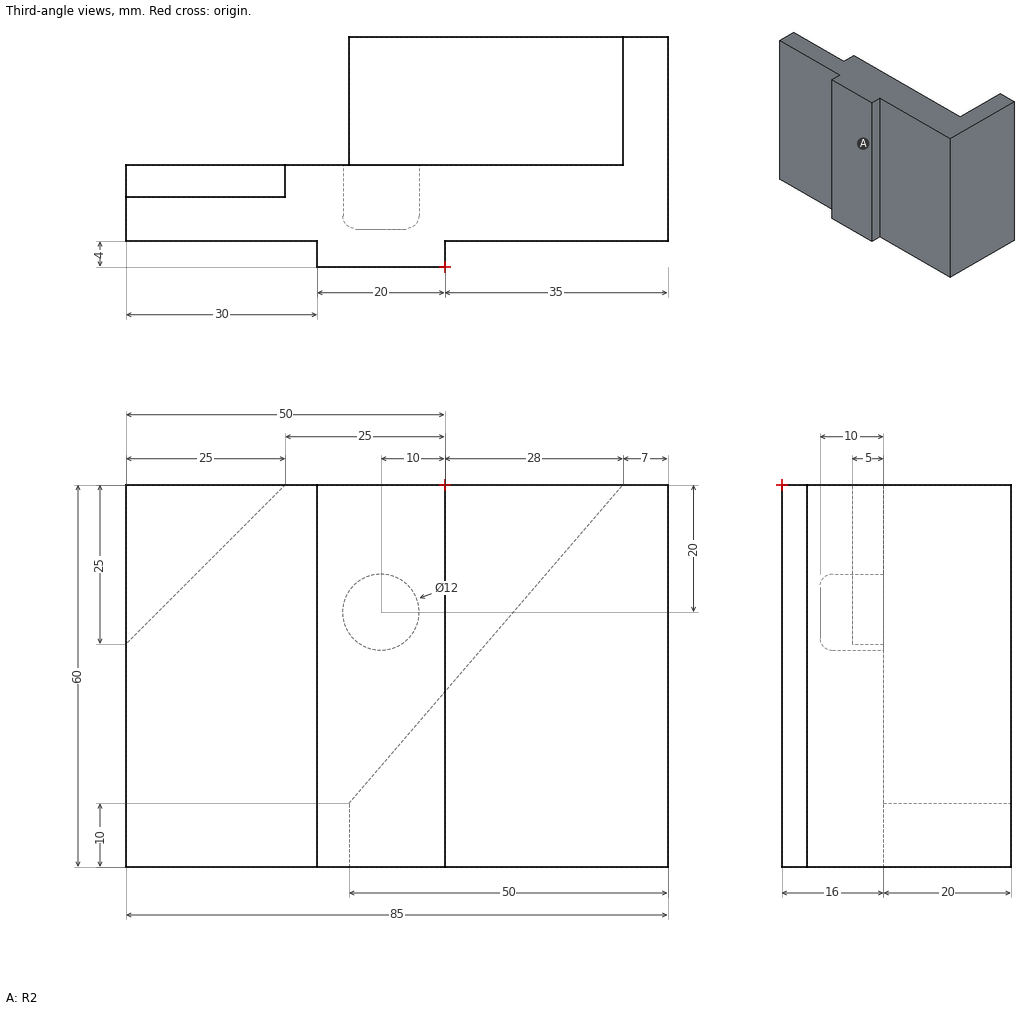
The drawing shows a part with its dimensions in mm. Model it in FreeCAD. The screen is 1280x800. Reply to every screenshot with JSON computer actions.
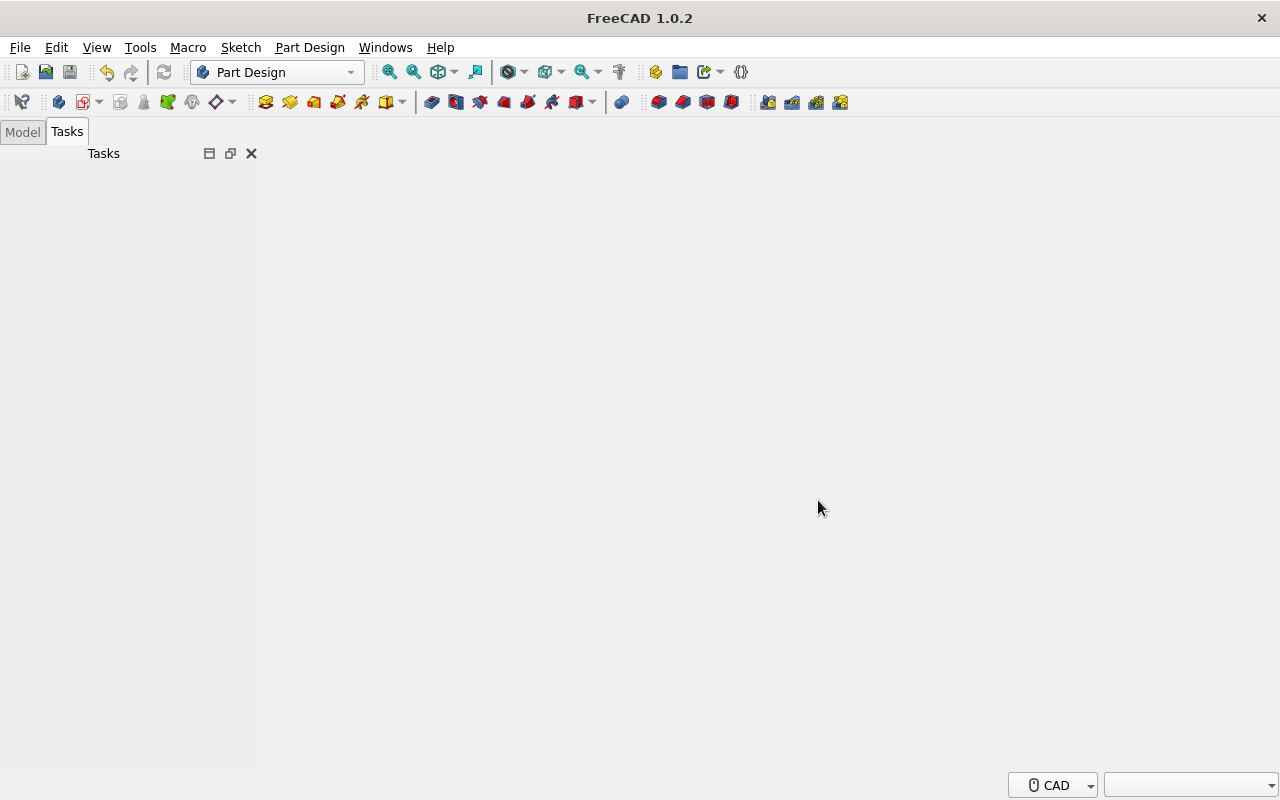
{"action": "left_click", "coordinate": [22, 72]}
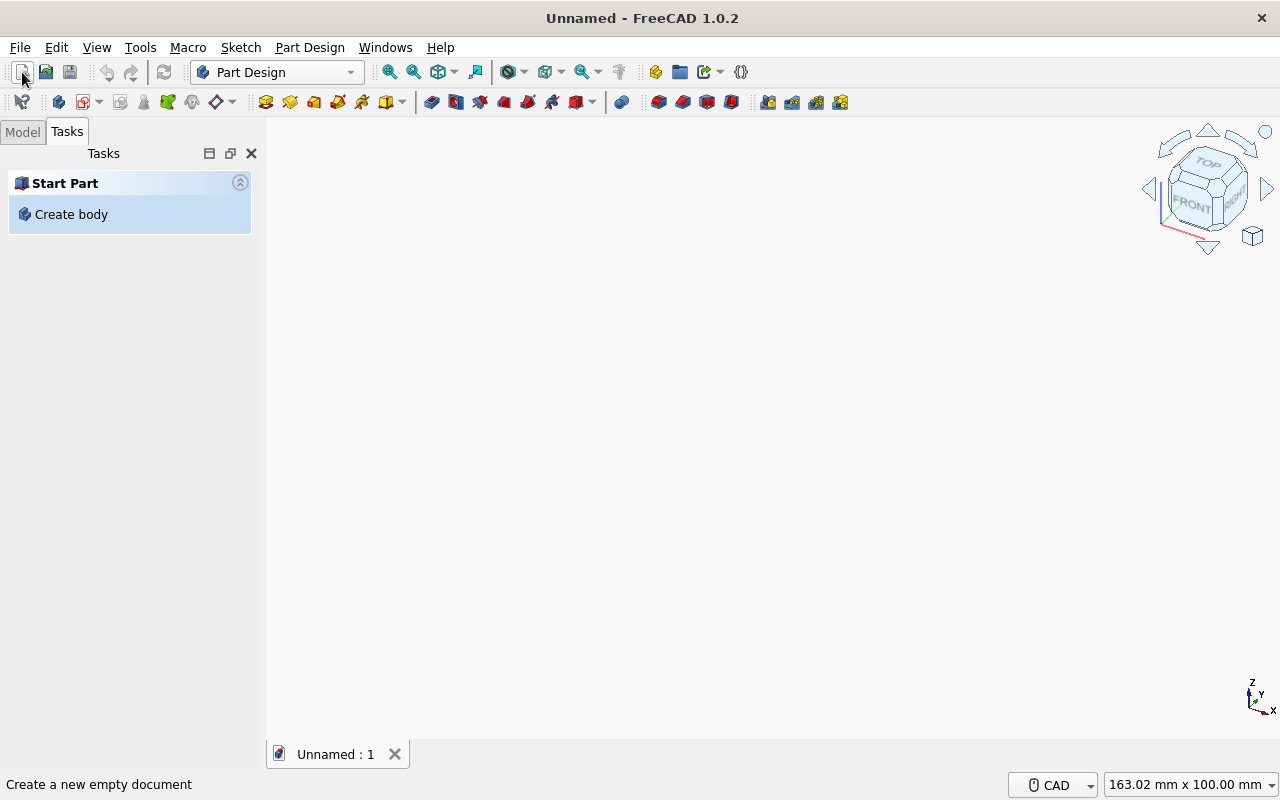
{"action": "left_click", "coordinate": [84, 102]}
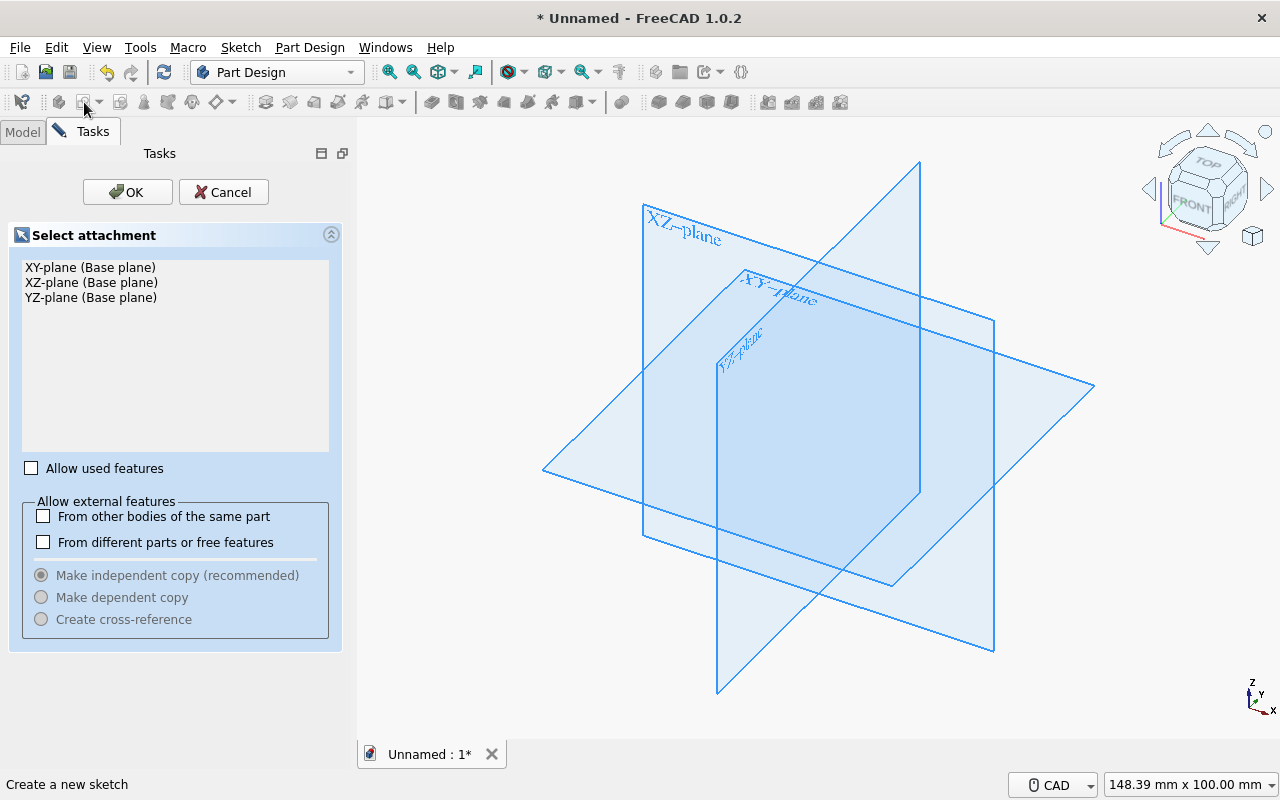
{"action": "left_click", "coordinate": [82, 282]}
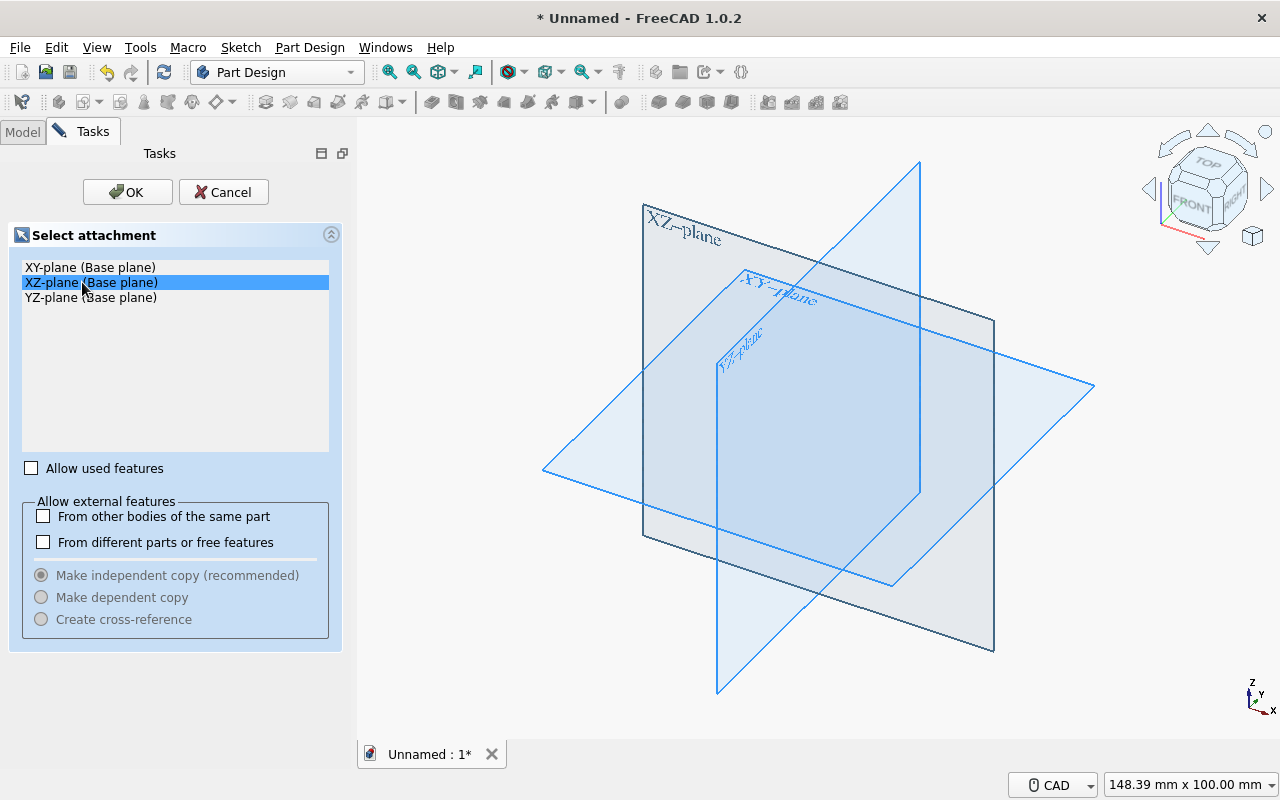
{"action": "left_click", "coordinate": [128, 192]}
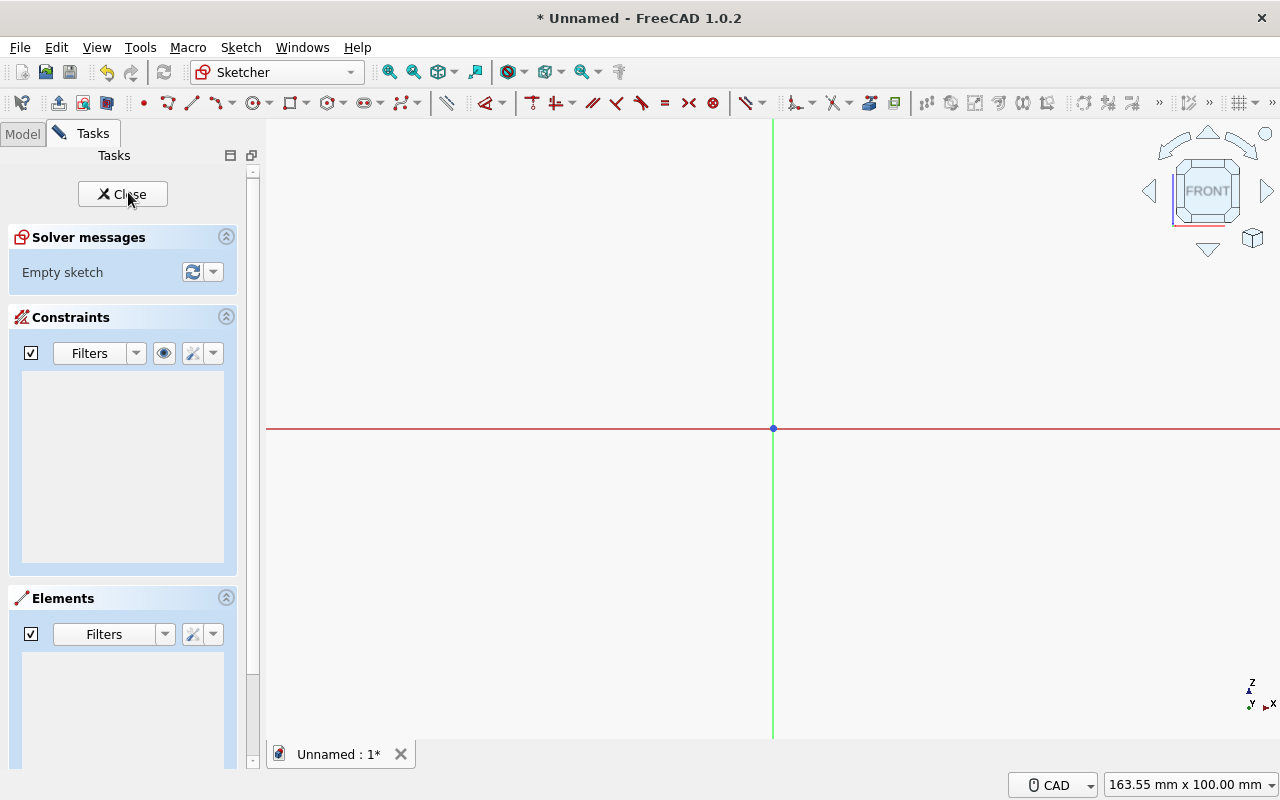
{"action": "scroll", "coordinate": [605, 147], "scroll_direction": "down", "scroll_amount": 1}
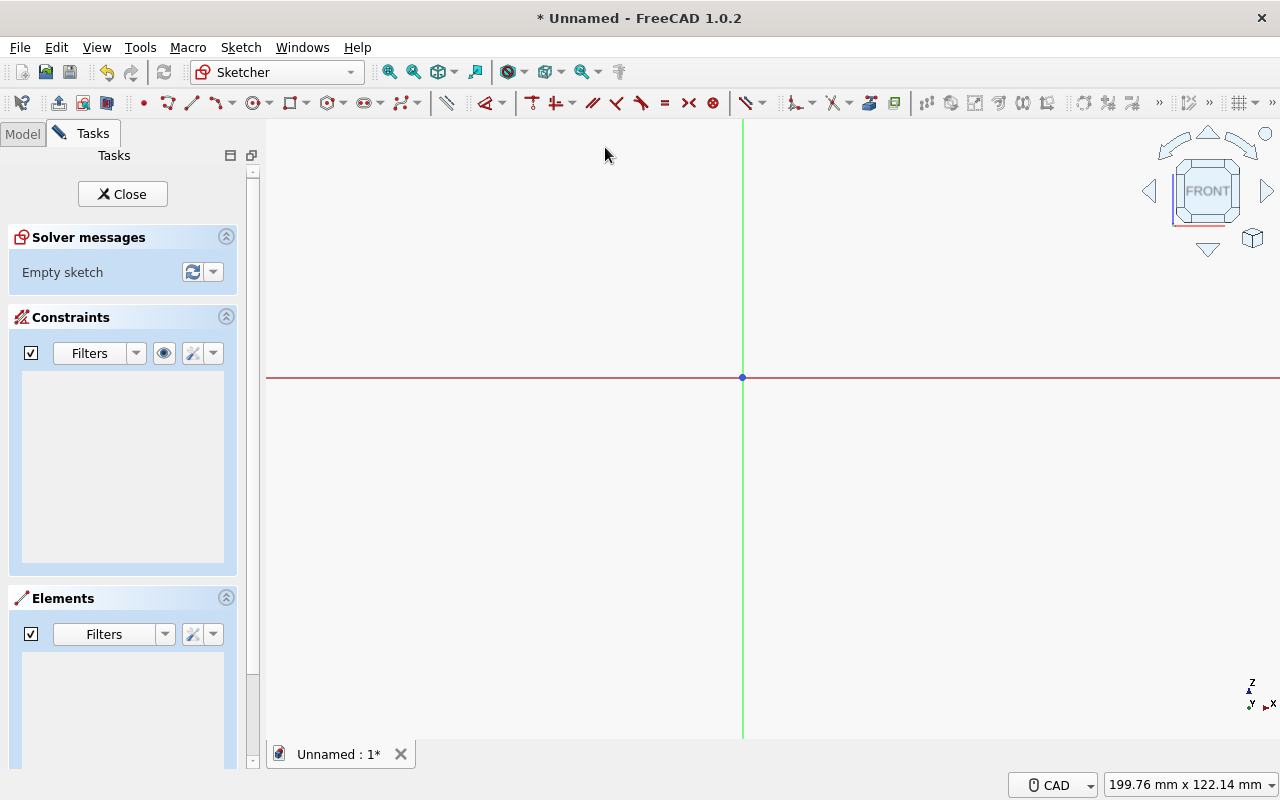
{"action": "left_click", "coordinate": [290, 104]}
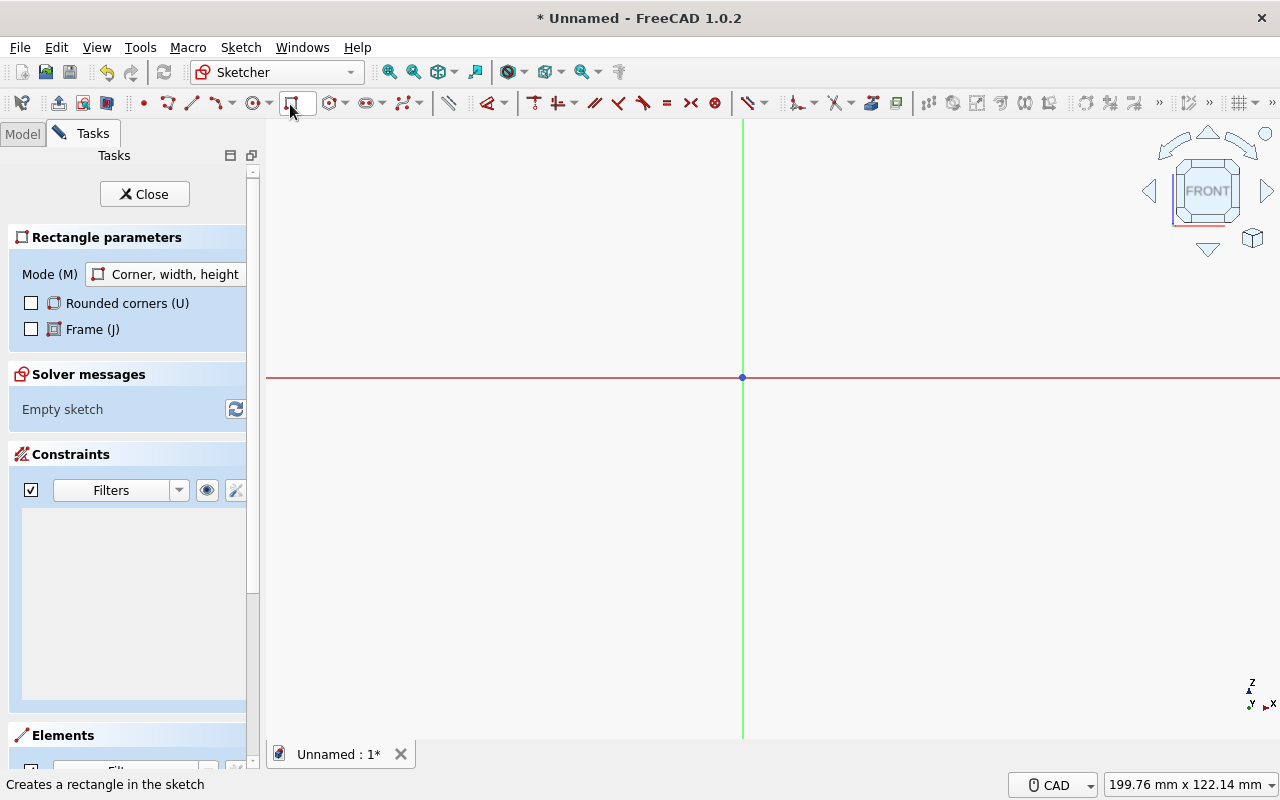
{"action": "left_click", "coordinate": [489, 378]}
{"action": "left_click", "coordinate": [920, 682]}
{"action": "key", "text": "Escape"}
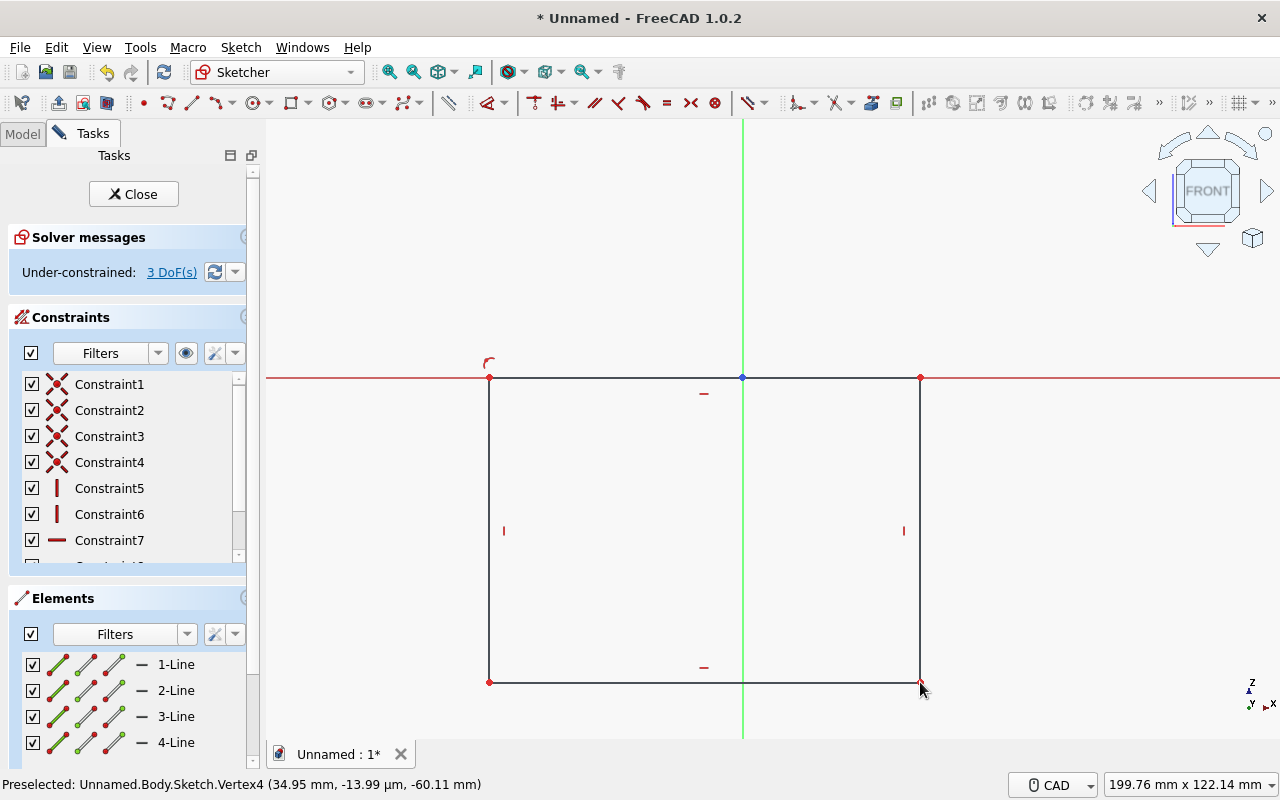
{"action": "left_click", "coordinate": [488, 104]}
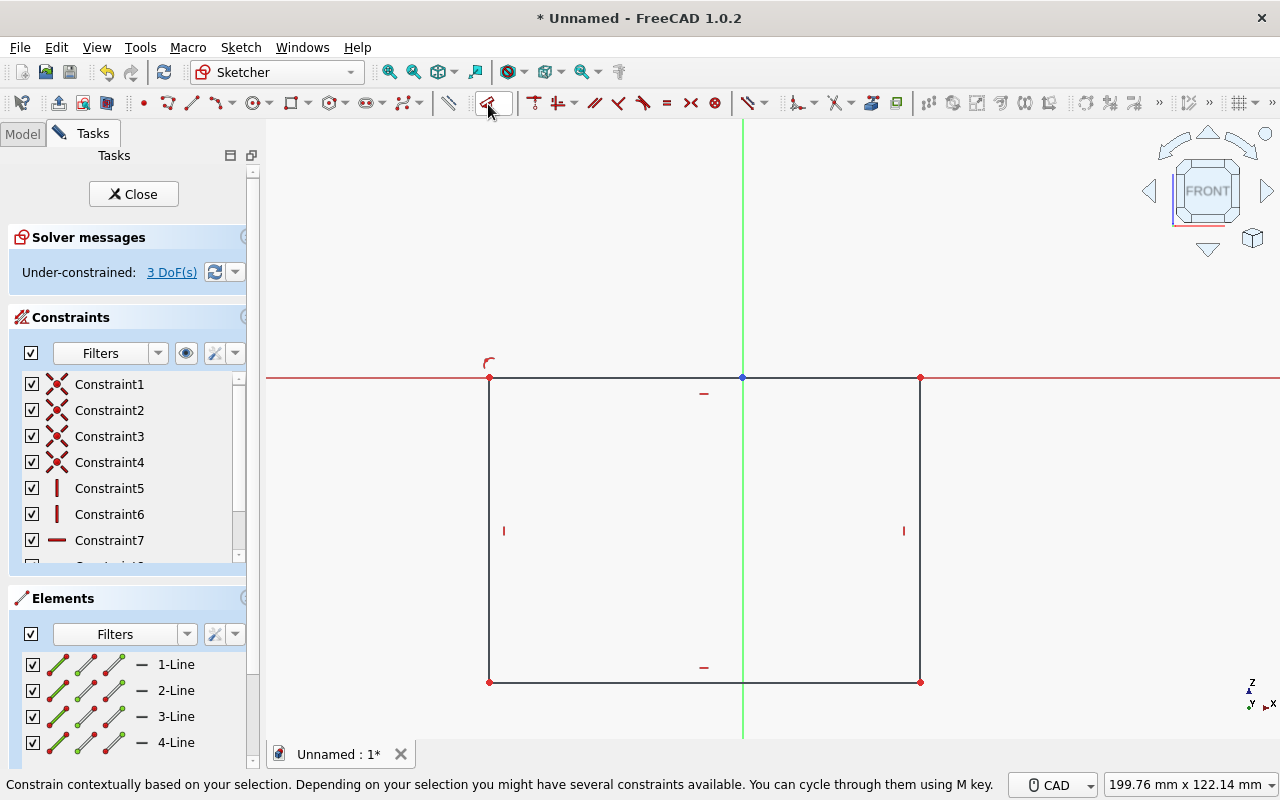
{"action": "left_click", "coordinate": [489, 469]}
{"action": "left_click", "coordinate": [455, 530]}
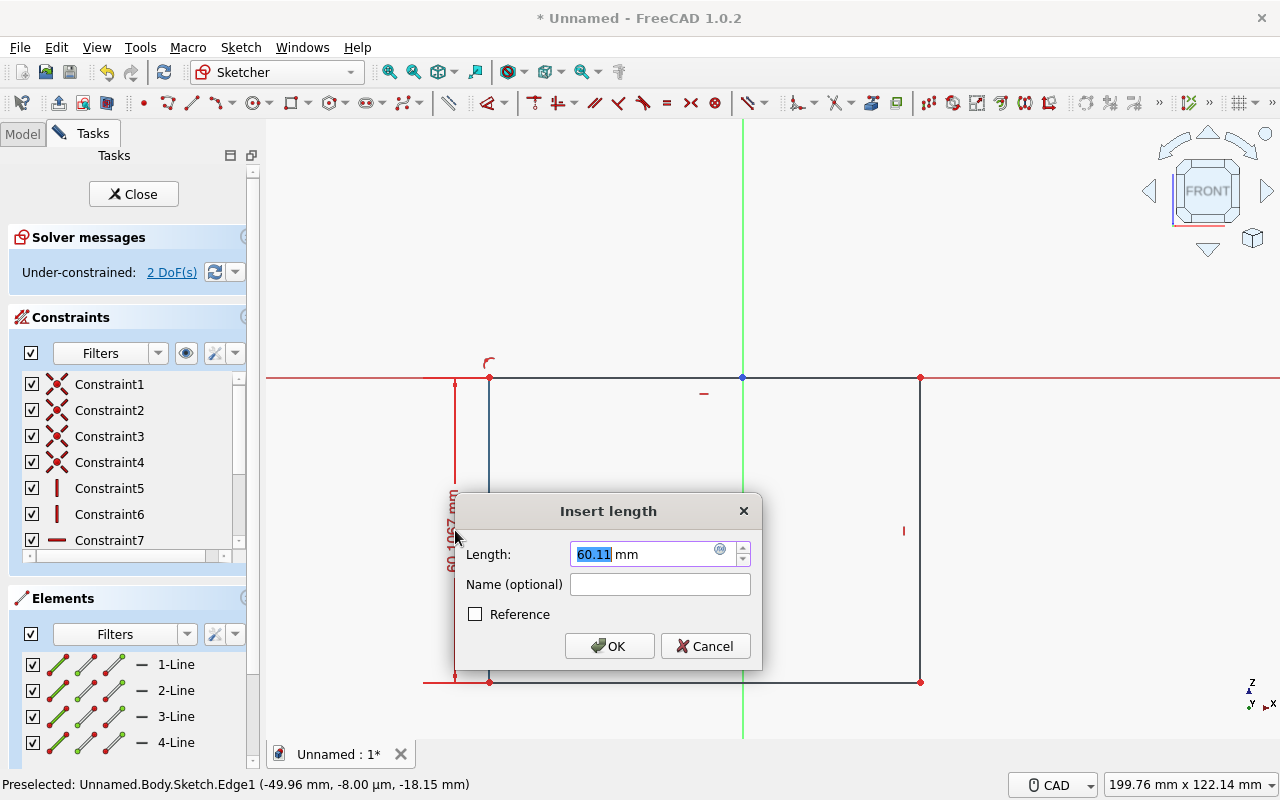
{"action": "type", "text": "60"}
{"action": "key", "text": "Return"}